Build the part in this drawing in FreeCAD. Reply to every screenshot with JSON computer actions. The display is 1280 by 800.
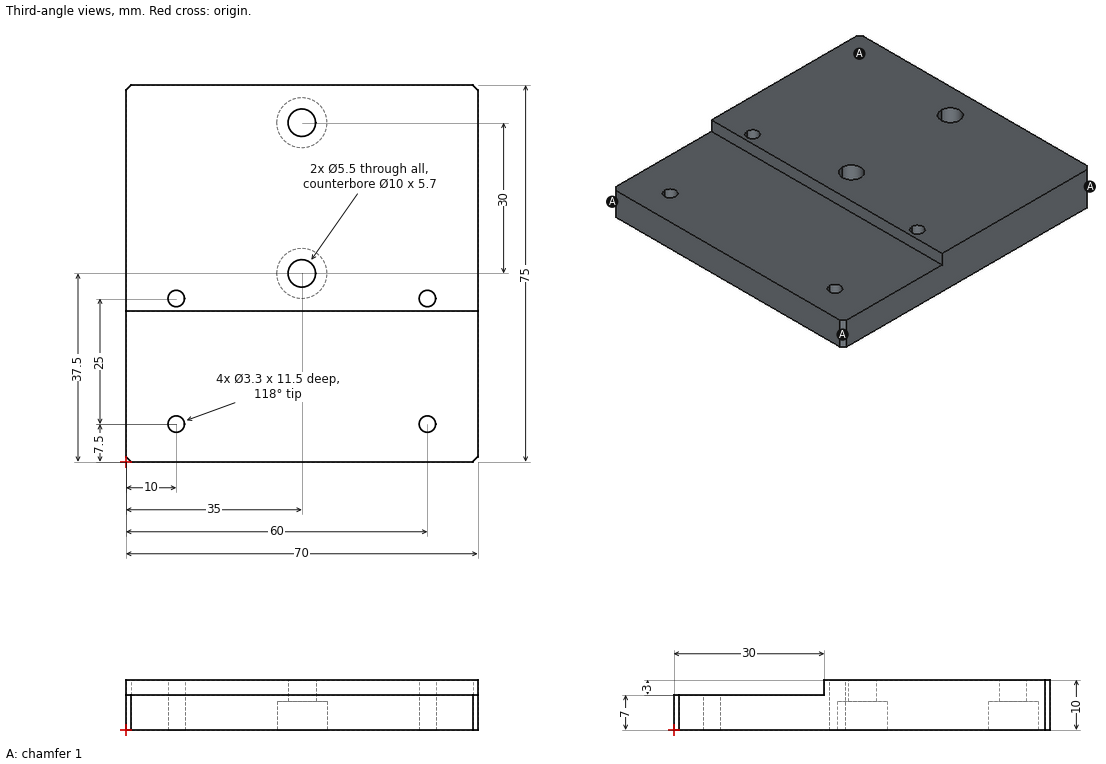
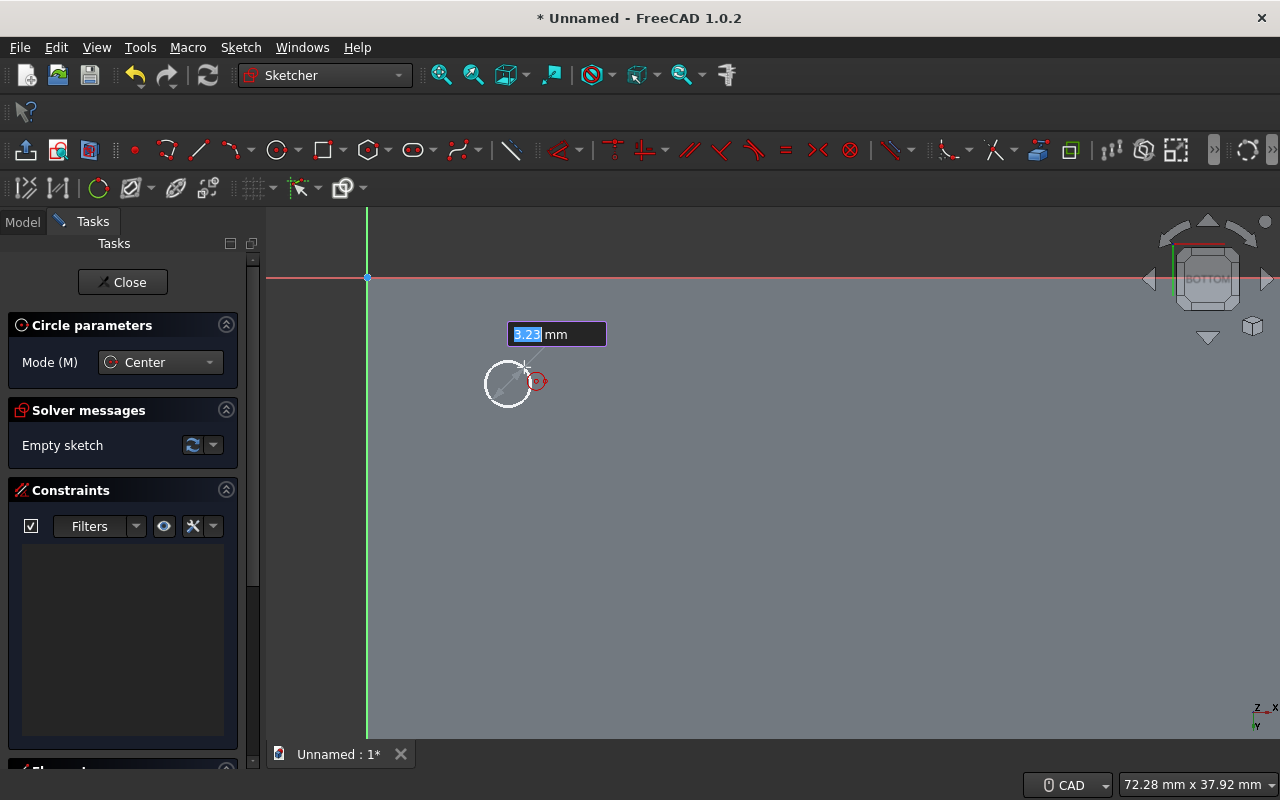
{"action": "type", "text": "3.3"}
{"action": "key", "text": "Return"}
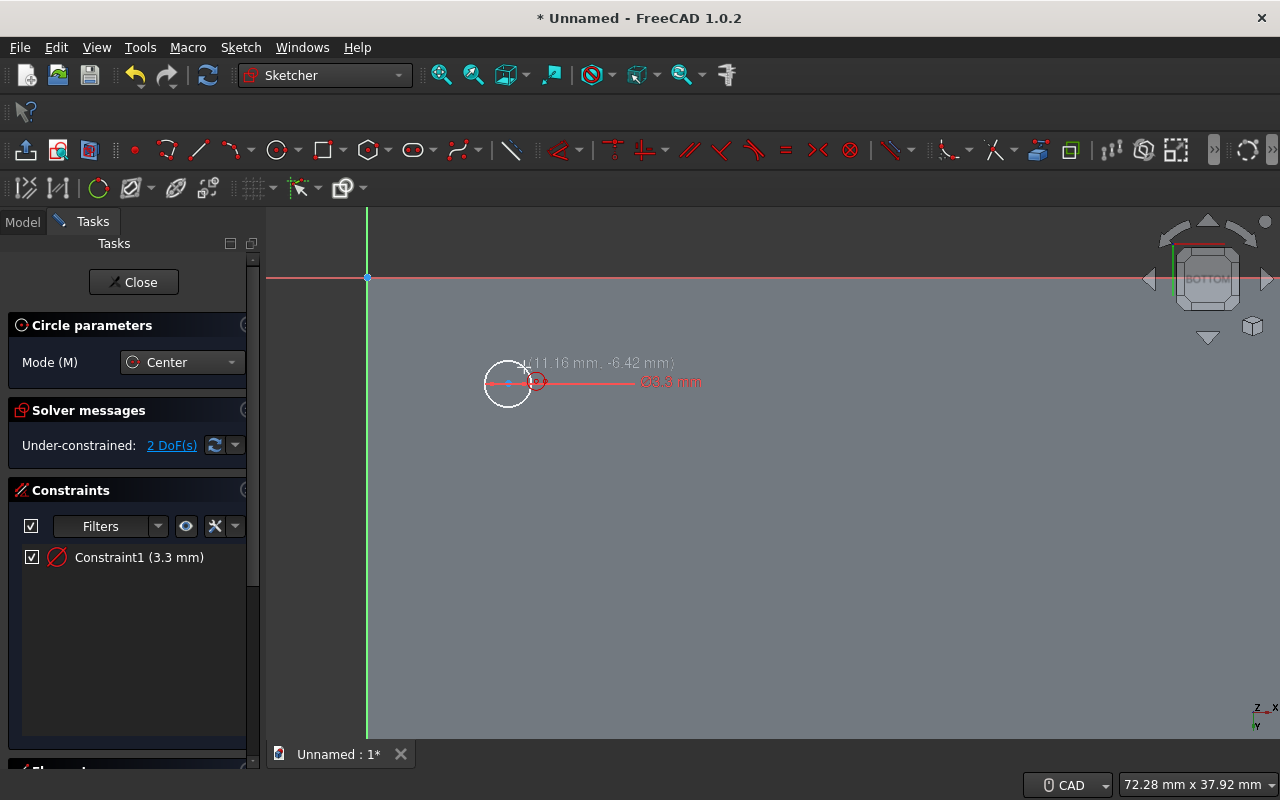
{"action": "scroll", "coordinate": [511, 383], "scroll_direction": "down", "scroll_amount": 2}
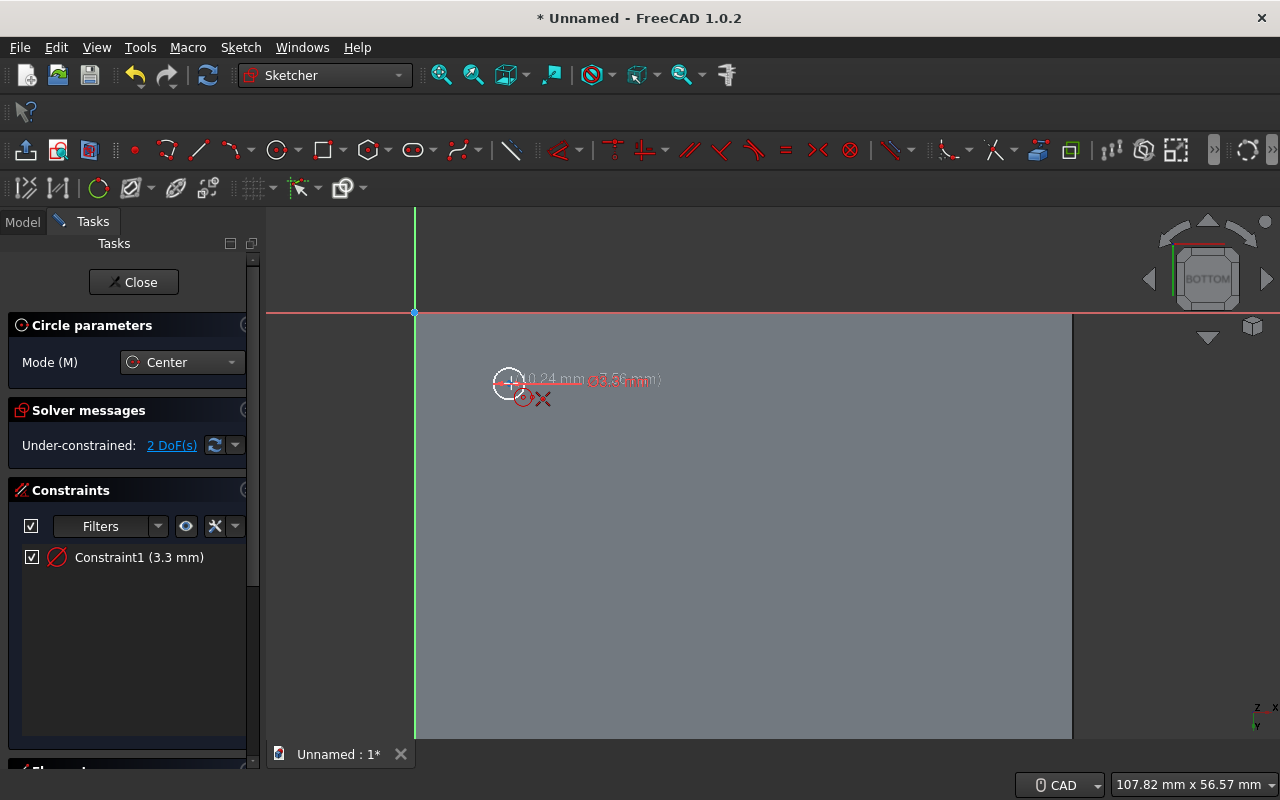
{"action": "scroll", "coordinate": [509, 618], "scroll_direction": "up", "scroll_amount": 2}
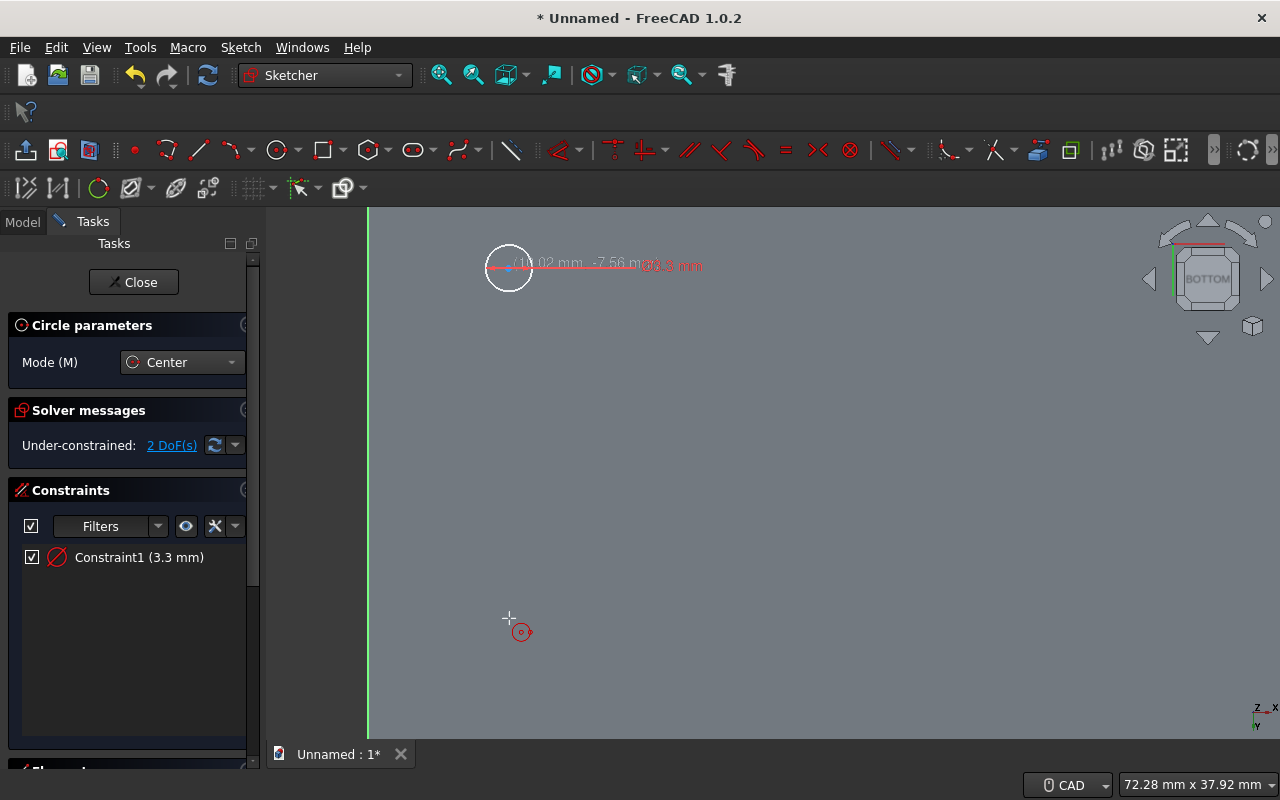
{"action": "left_click", "coordinate": [509, 618]}
{"action": "mouse_move", "coordinate": [525, 602]}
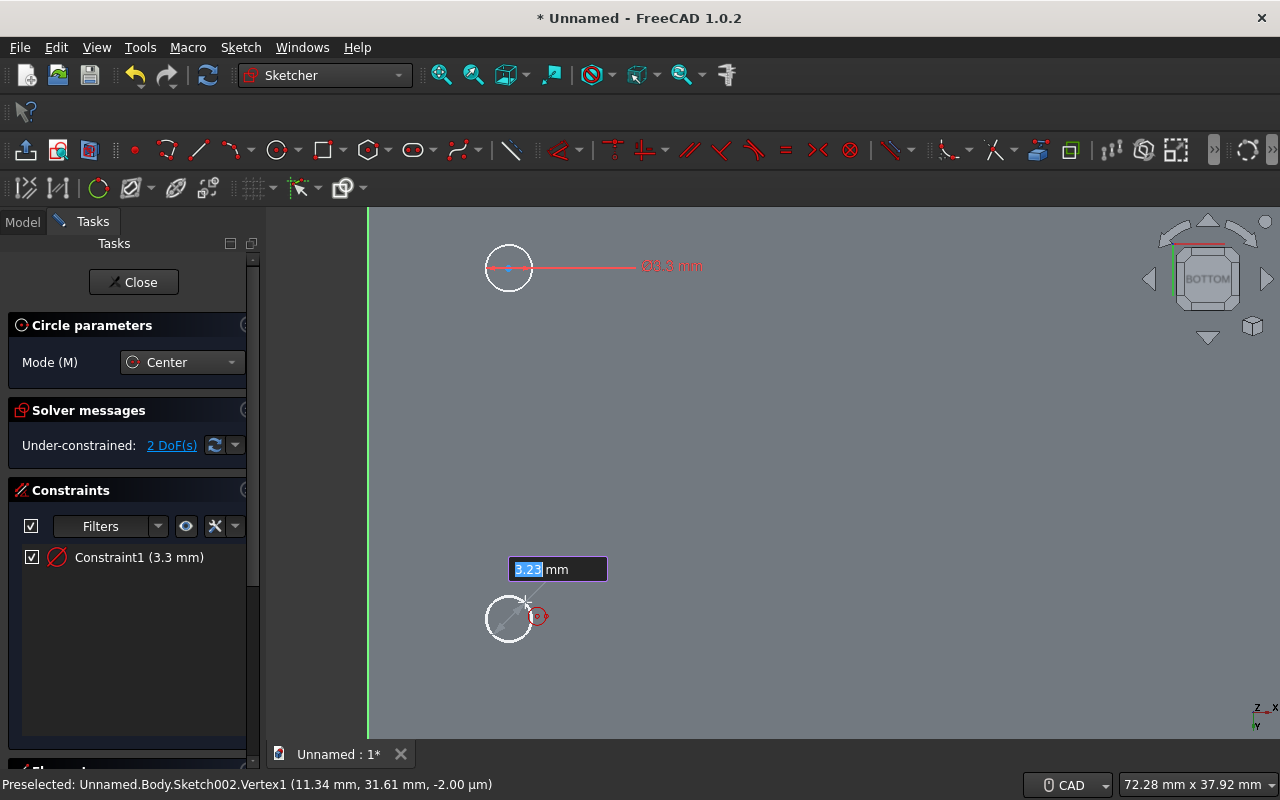
{"action": "type", "text": "3.3"}
{"action": "key", "text": "Return"}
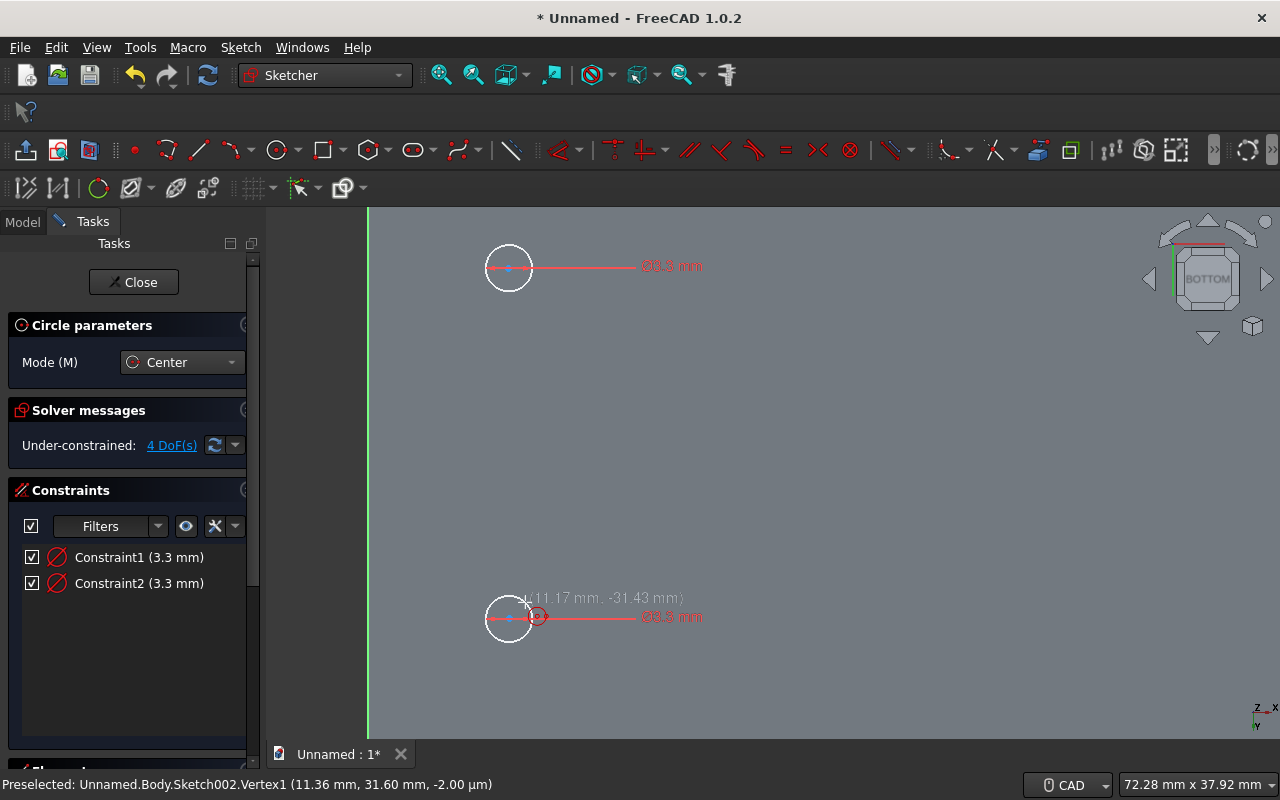
{"action": "scroll", "coordinate": [509, 618], "scroll_direction": "down", "scroll_amount": 2}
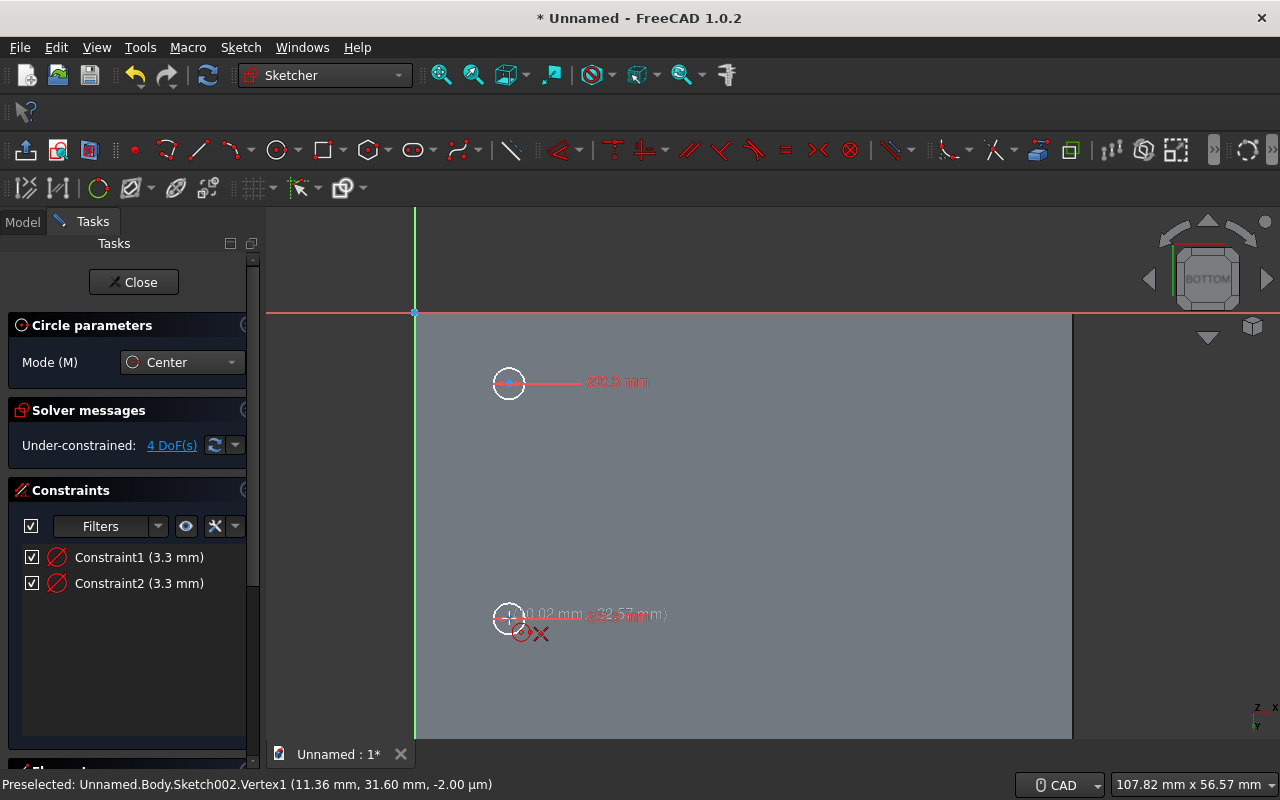
{"action": "scroll", "coordinate": [979, 383], "scroll_direction": "up", "scroll_amount": 2}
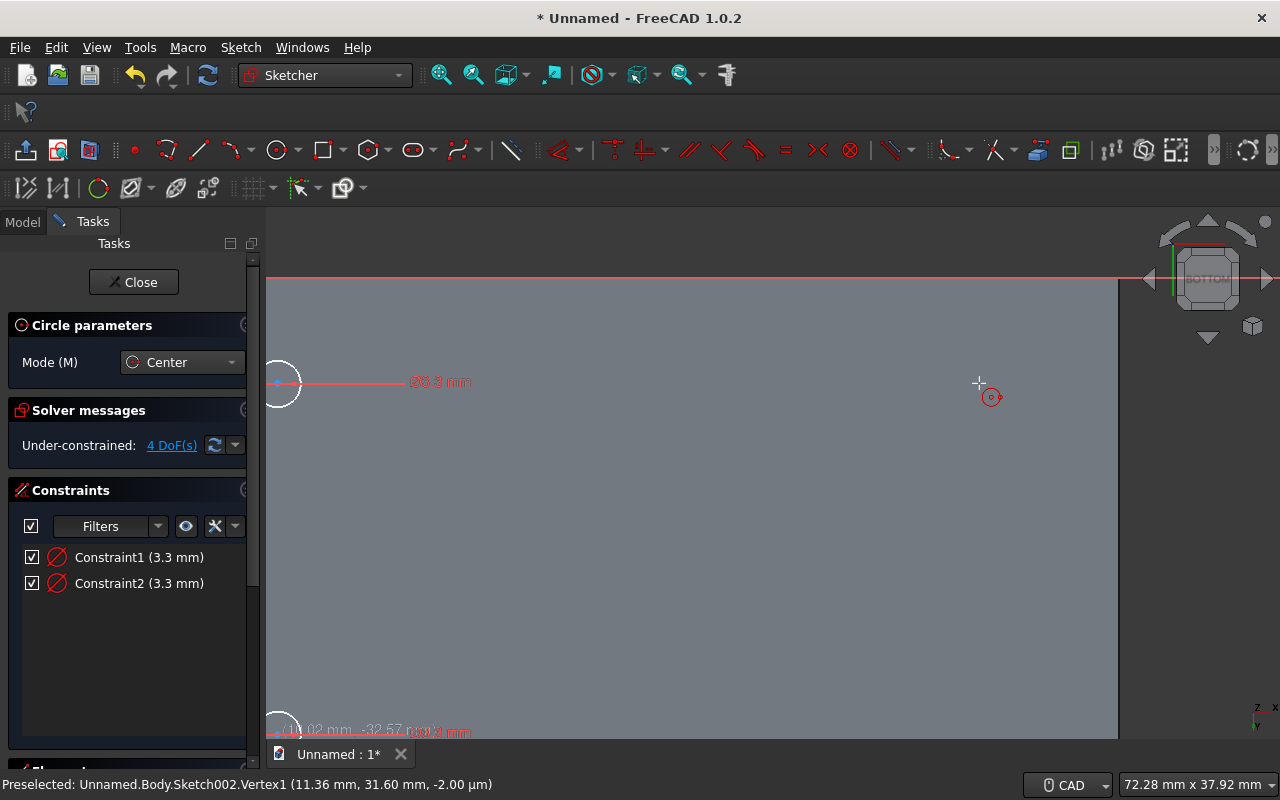
{"action": "left_click", "coordinate": [979, 383]}
{"action": "mouse_move", "coordinate": [995, 367]}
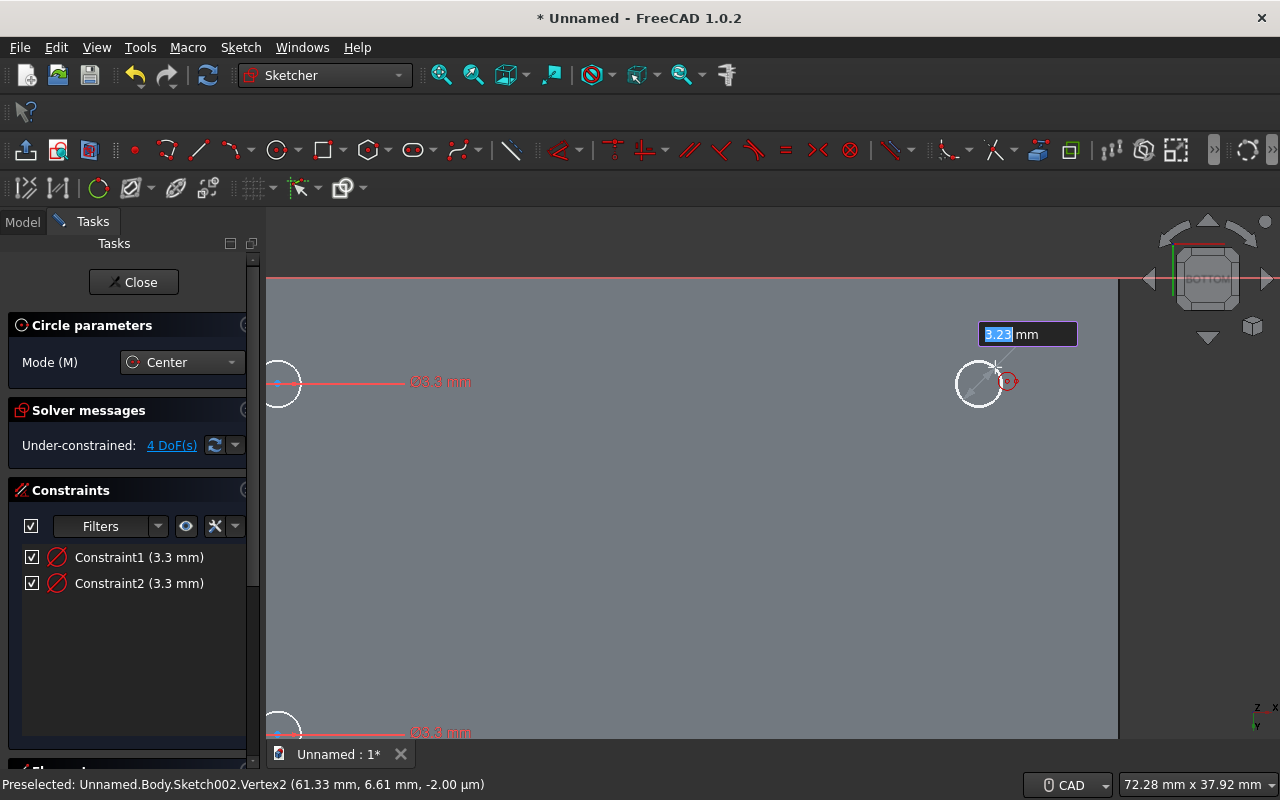
{"action": "type", "text": "3.3"}
{"action": "key", "text": "Return"}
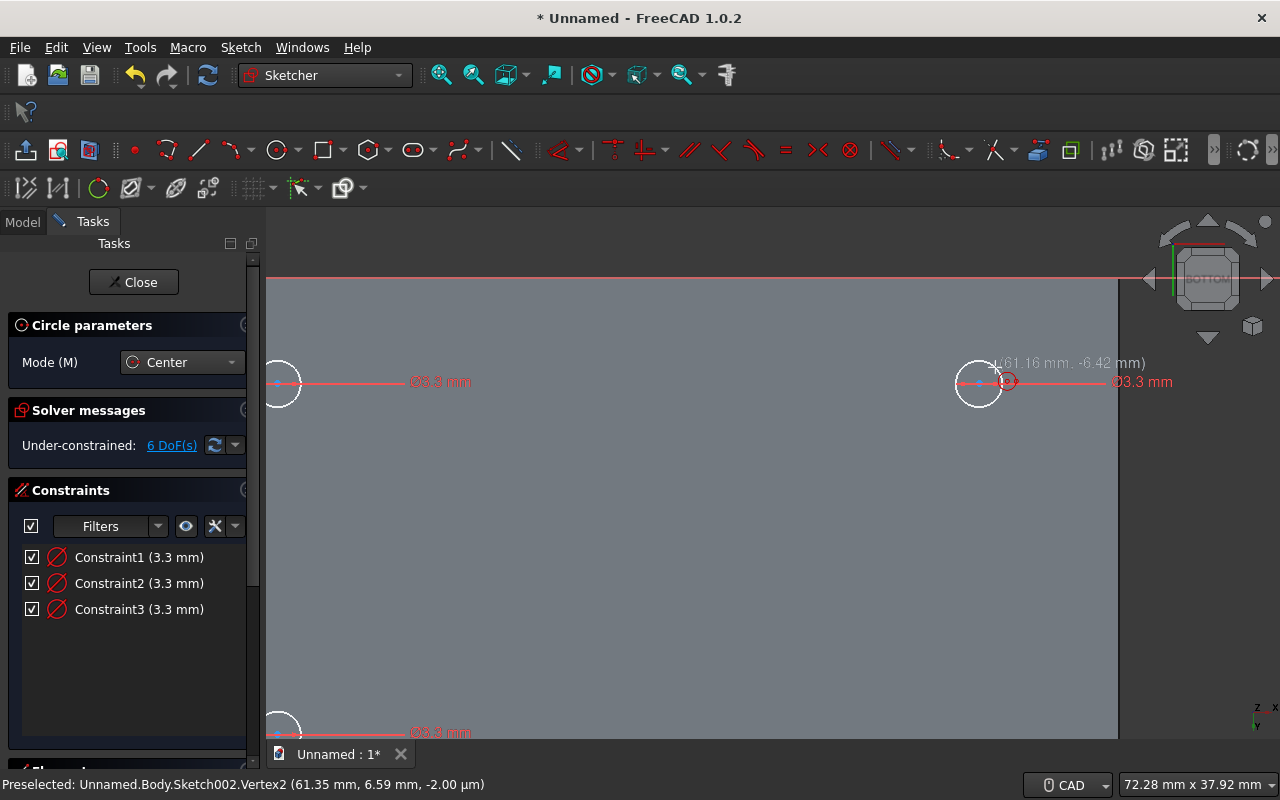
{"action": "scroll", "coordinate": [979, 383], "scroll_direction": "down", "scroll_amount": 2}